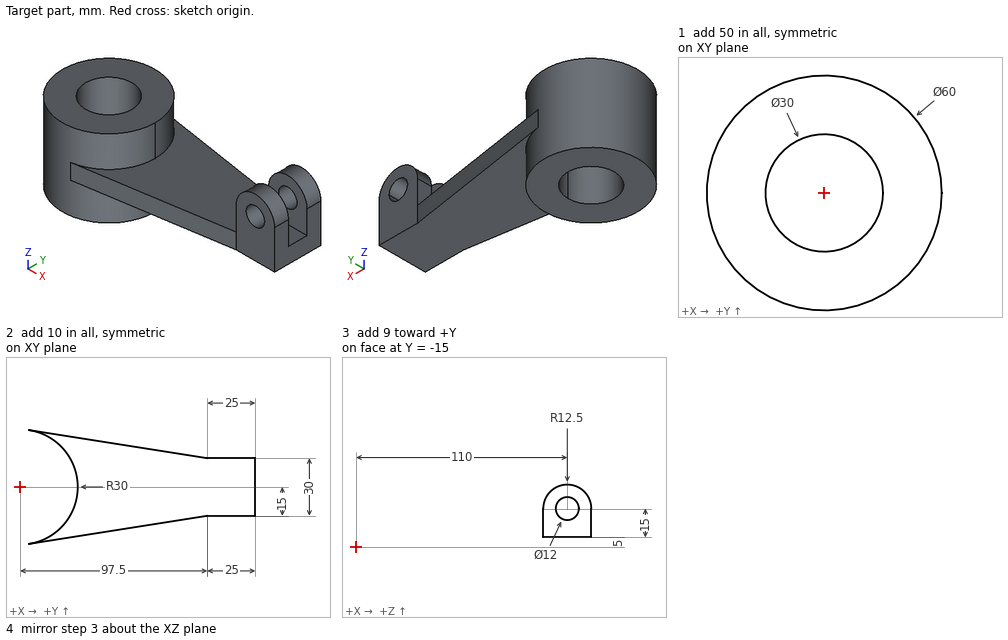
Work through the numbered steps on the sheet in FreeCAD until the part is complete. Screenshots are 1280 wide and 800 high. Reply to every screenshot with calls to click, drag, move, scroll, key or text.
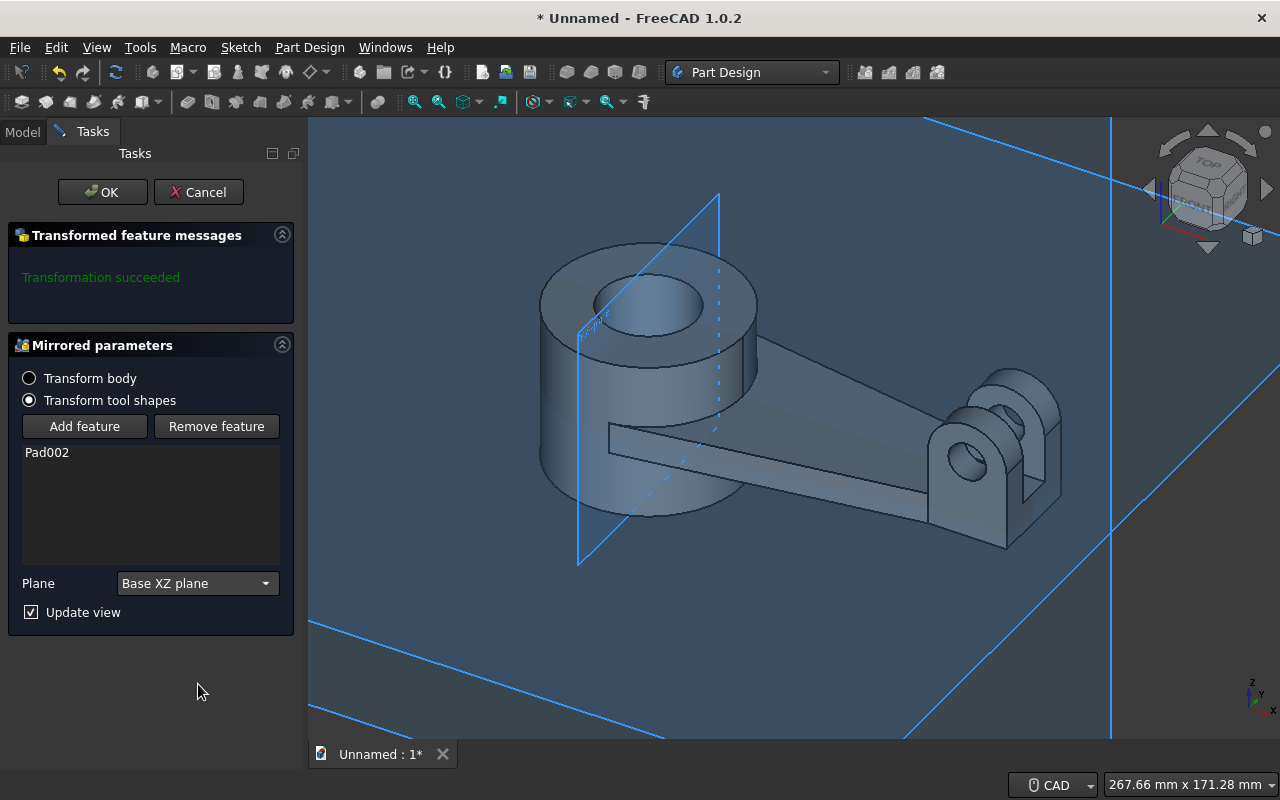
click(103, 192)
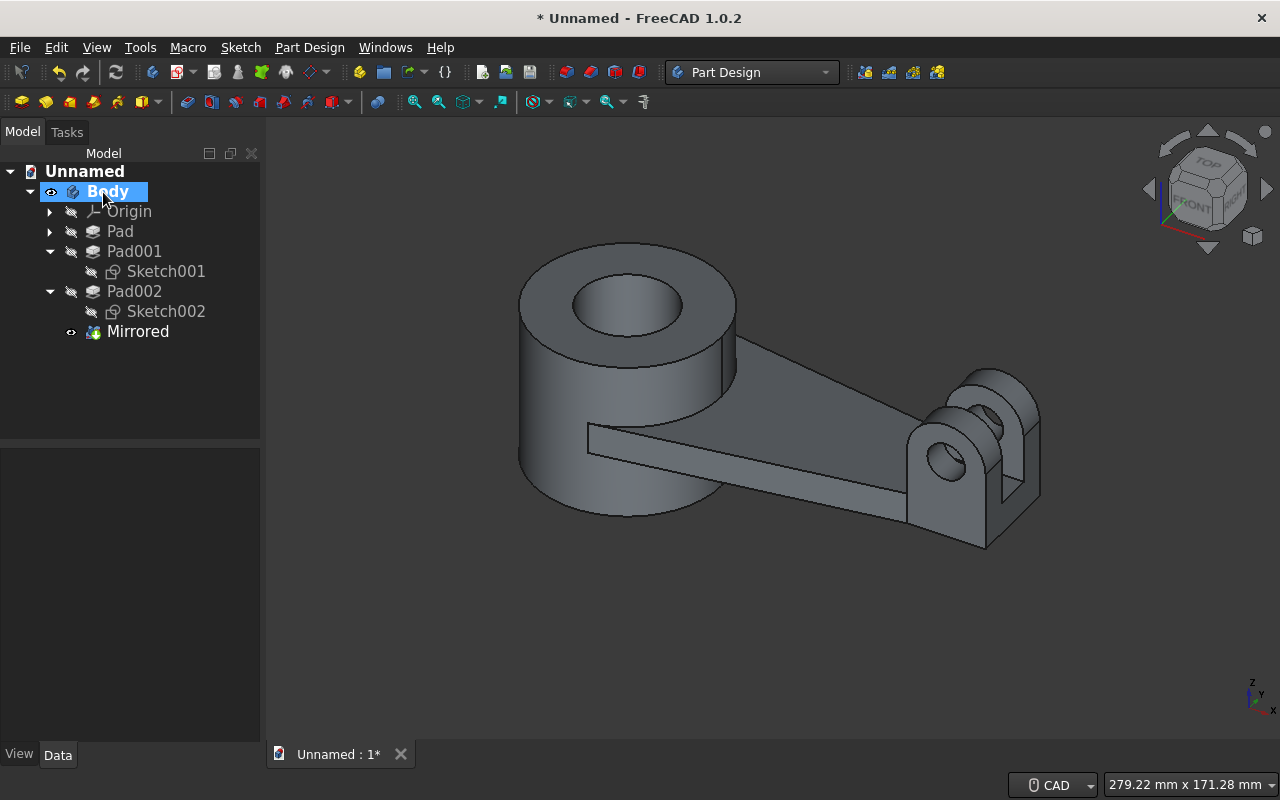
key(0)